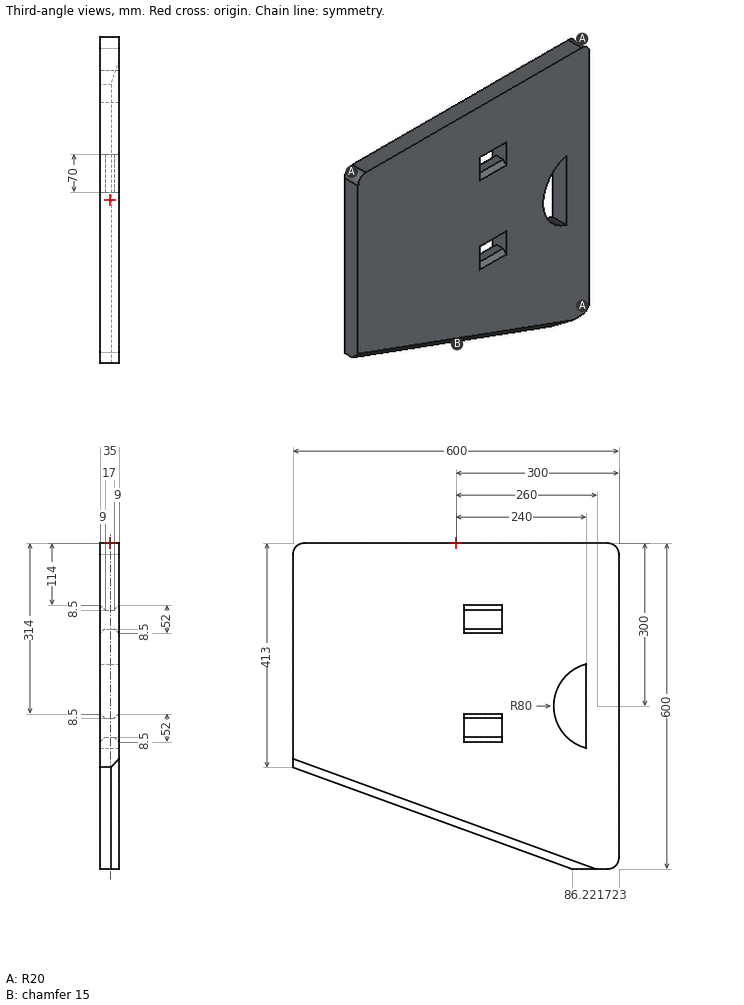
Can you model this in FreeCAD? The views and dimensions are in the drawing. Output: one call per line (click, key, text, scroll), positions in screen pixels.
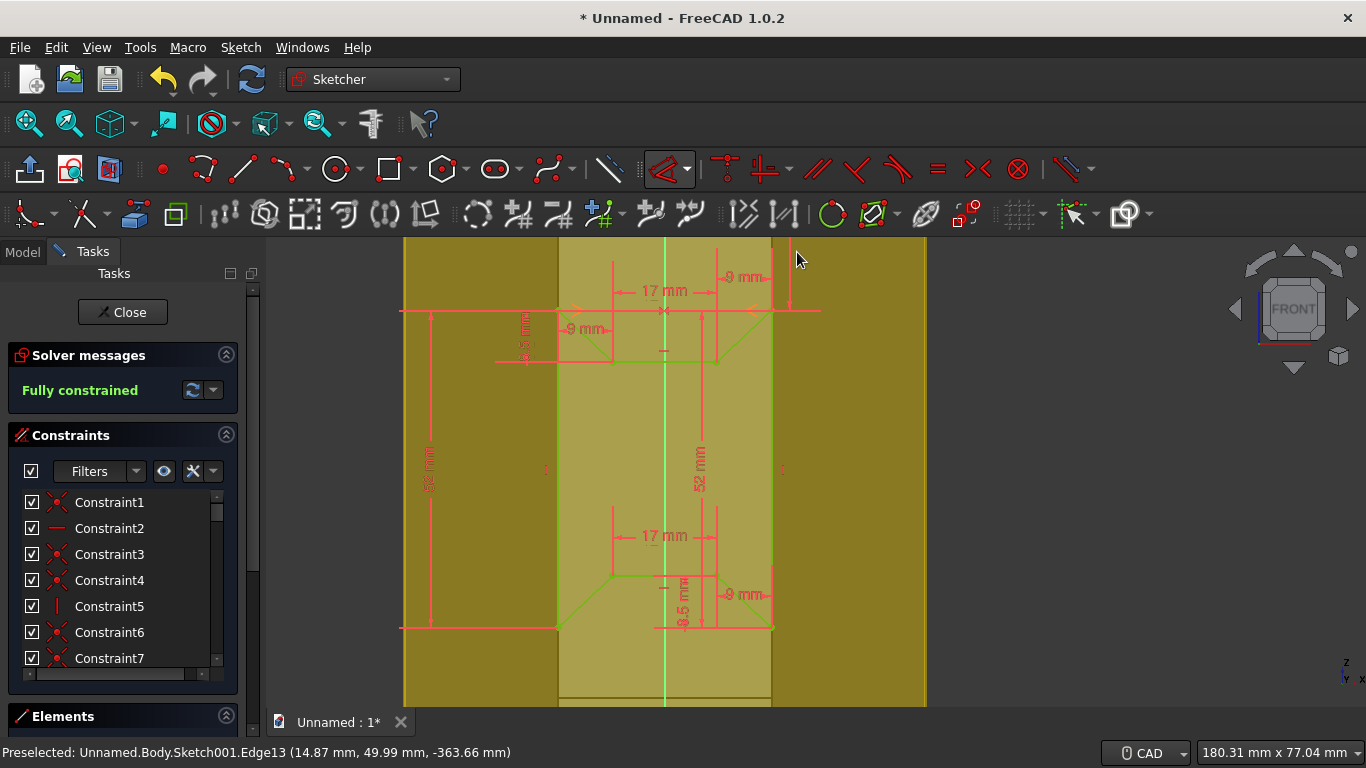
click(123, 312)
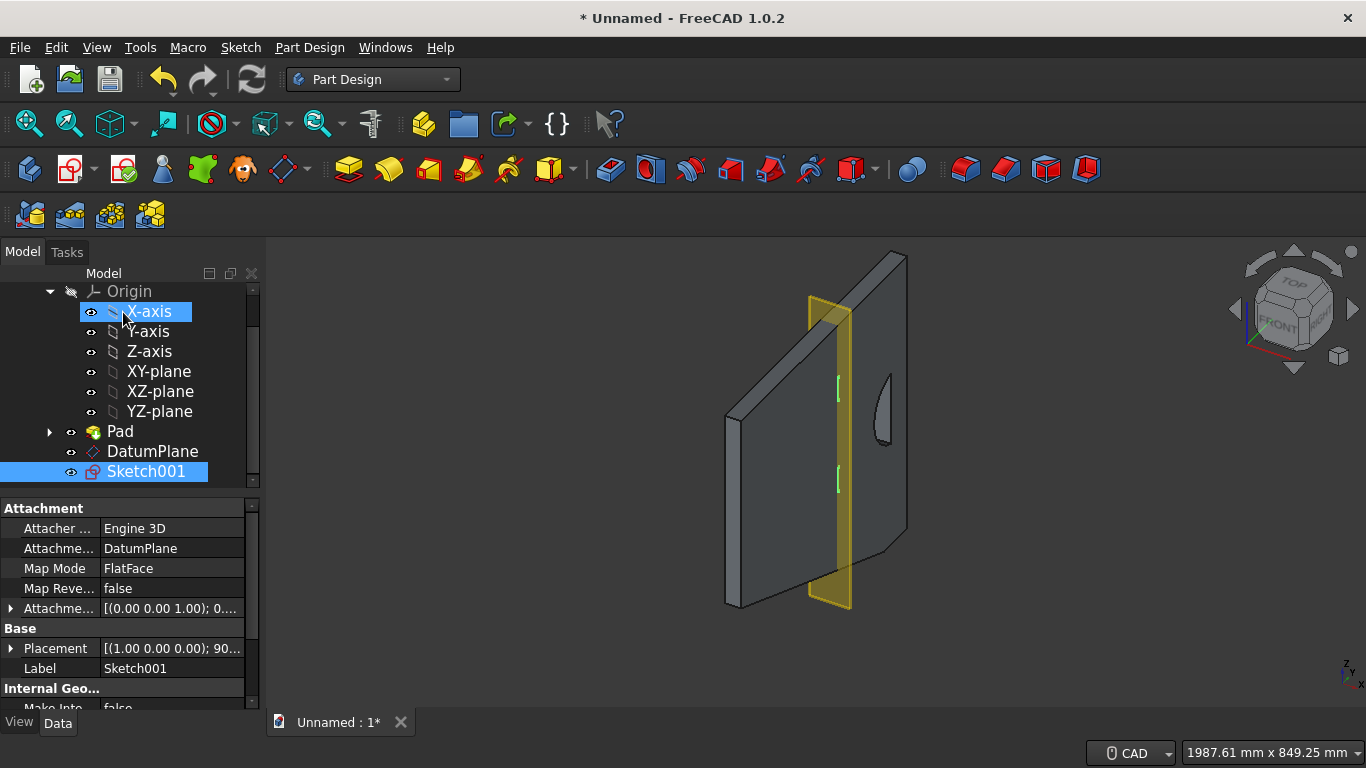
click(612, 170)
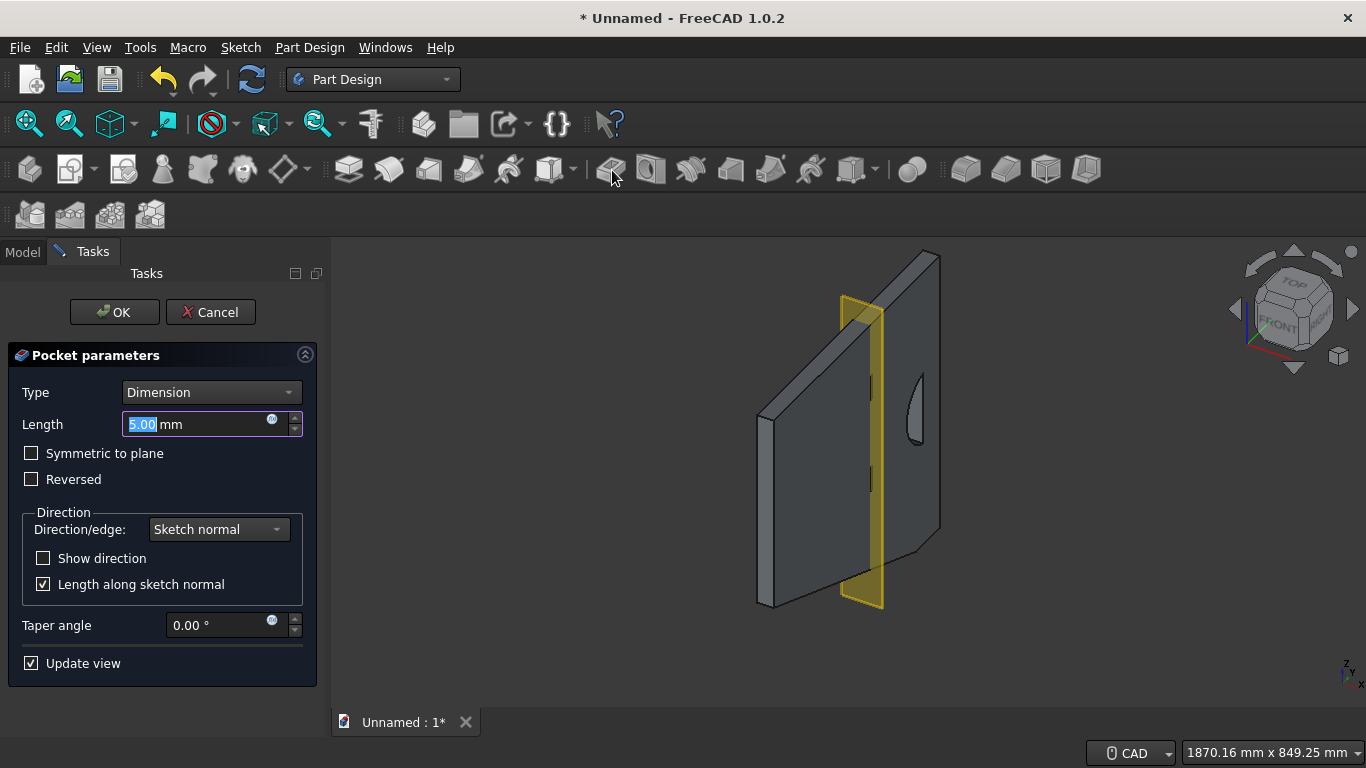
text(70)
key(Tab)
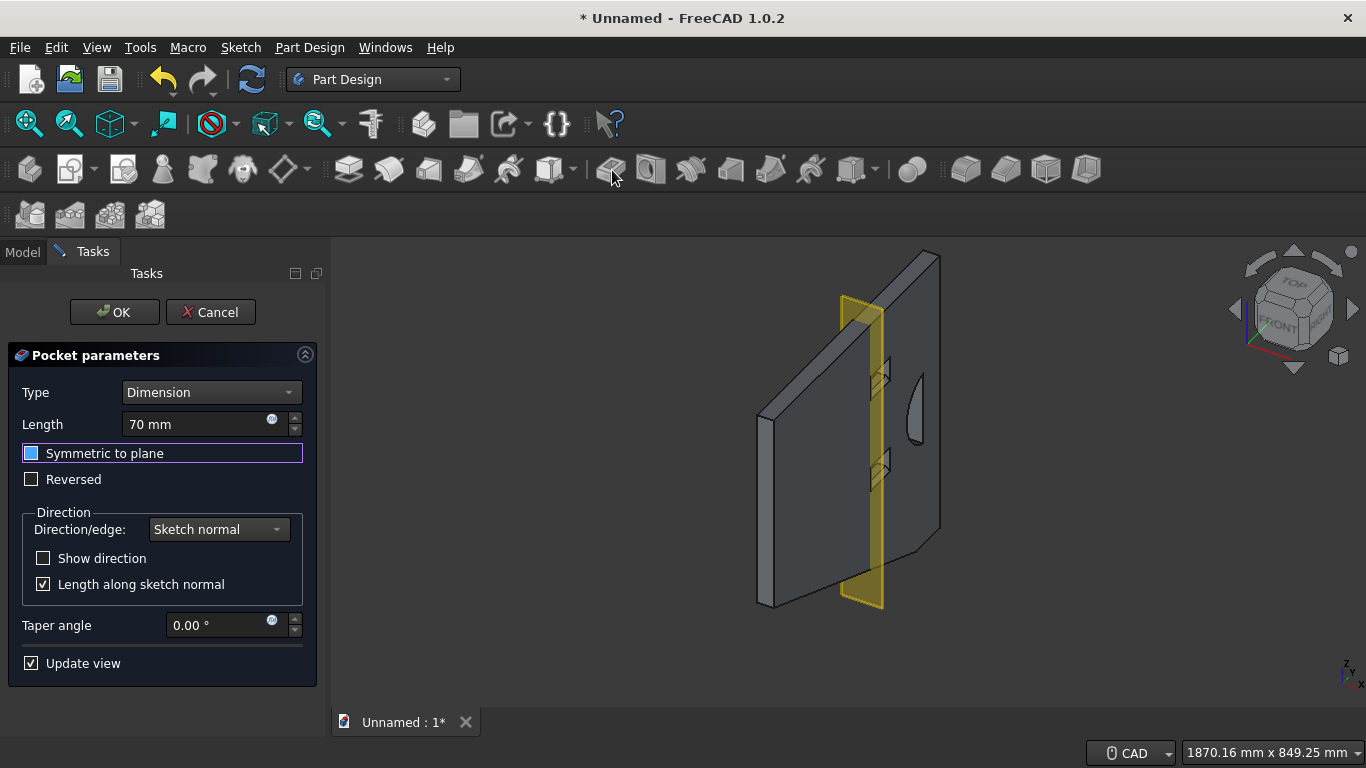
click(30, 453)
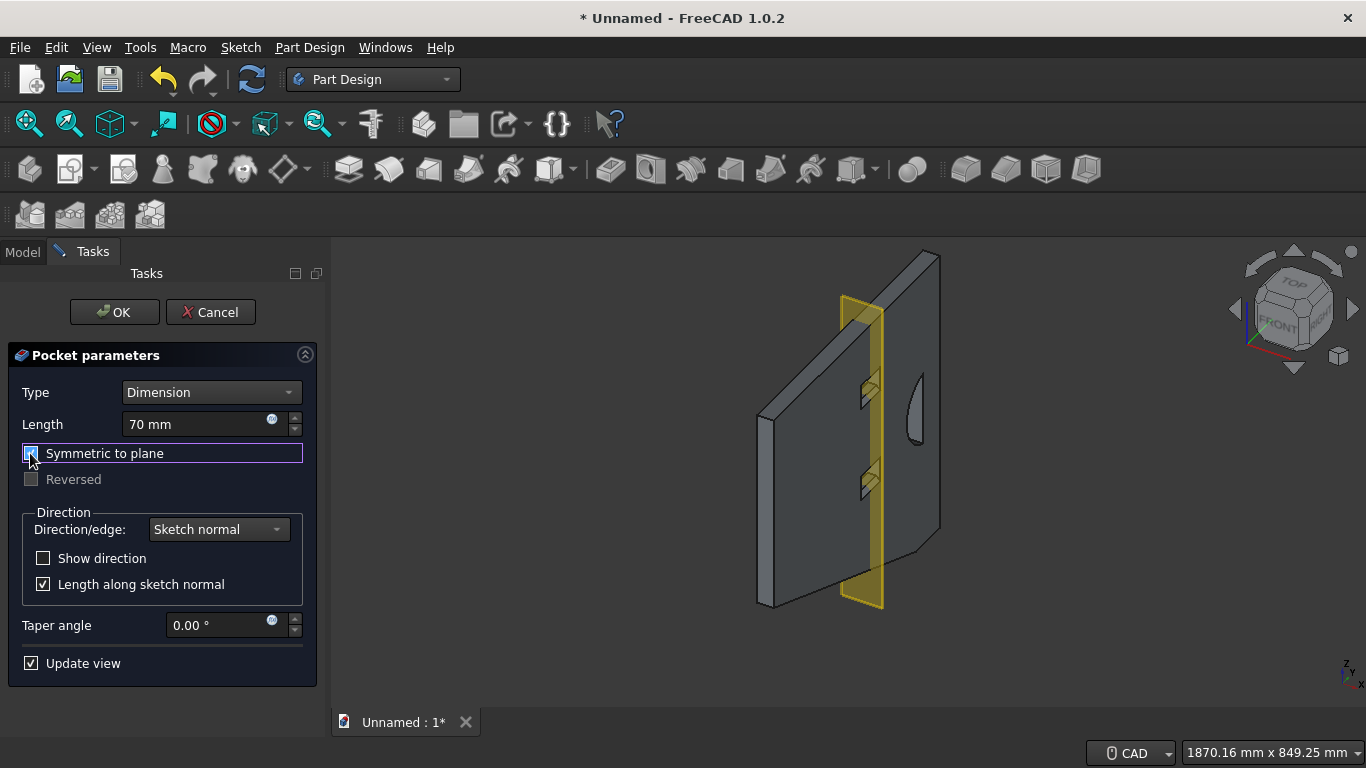
click(115, 312)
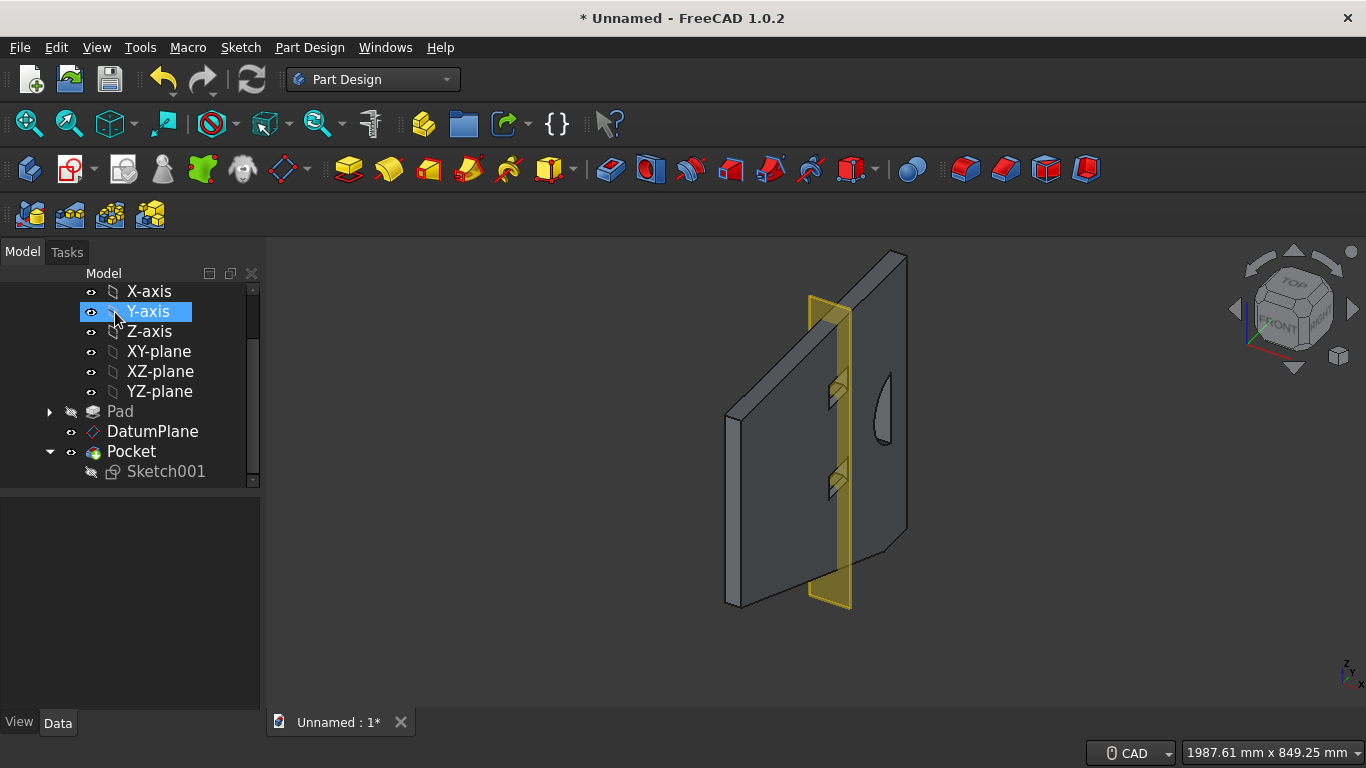
click(116, 432)
key(space)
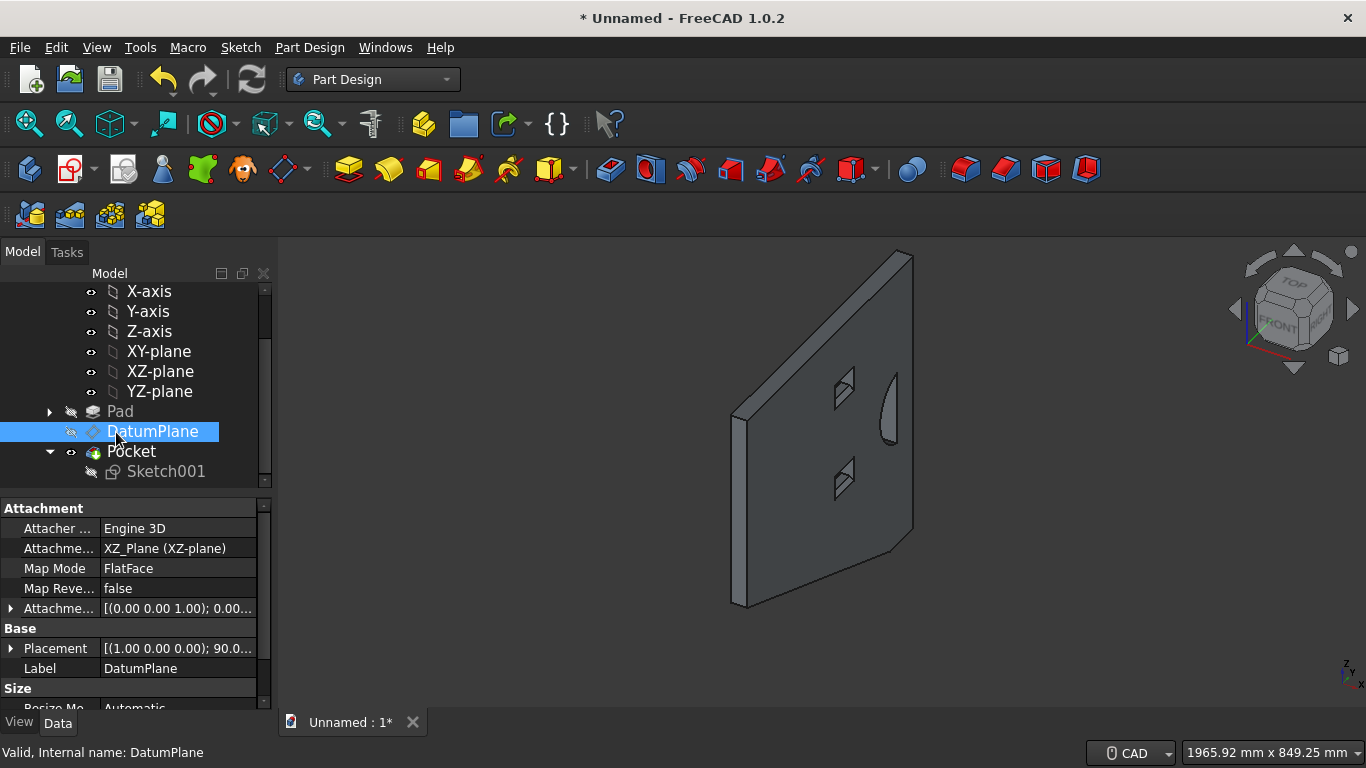
click(739, 417)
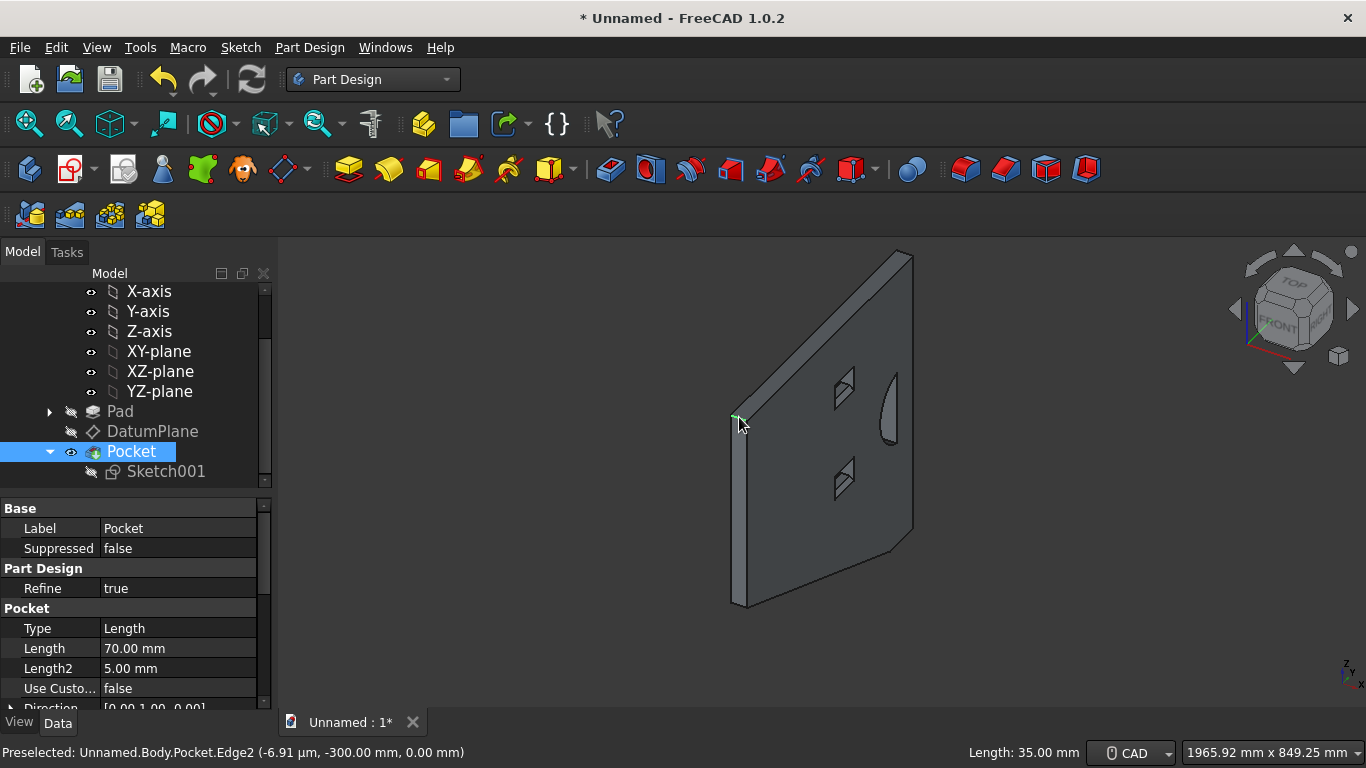
key(0)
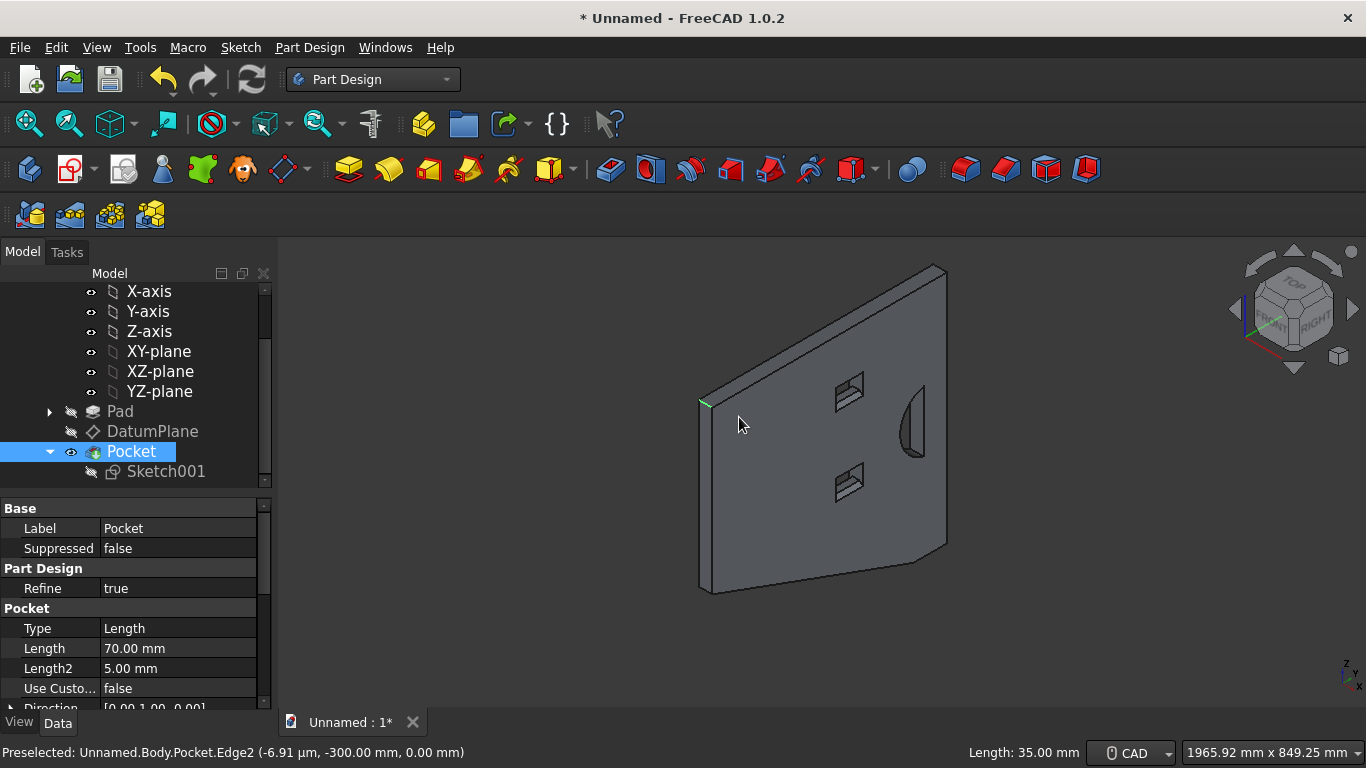
scroll(940, 267, up, 4)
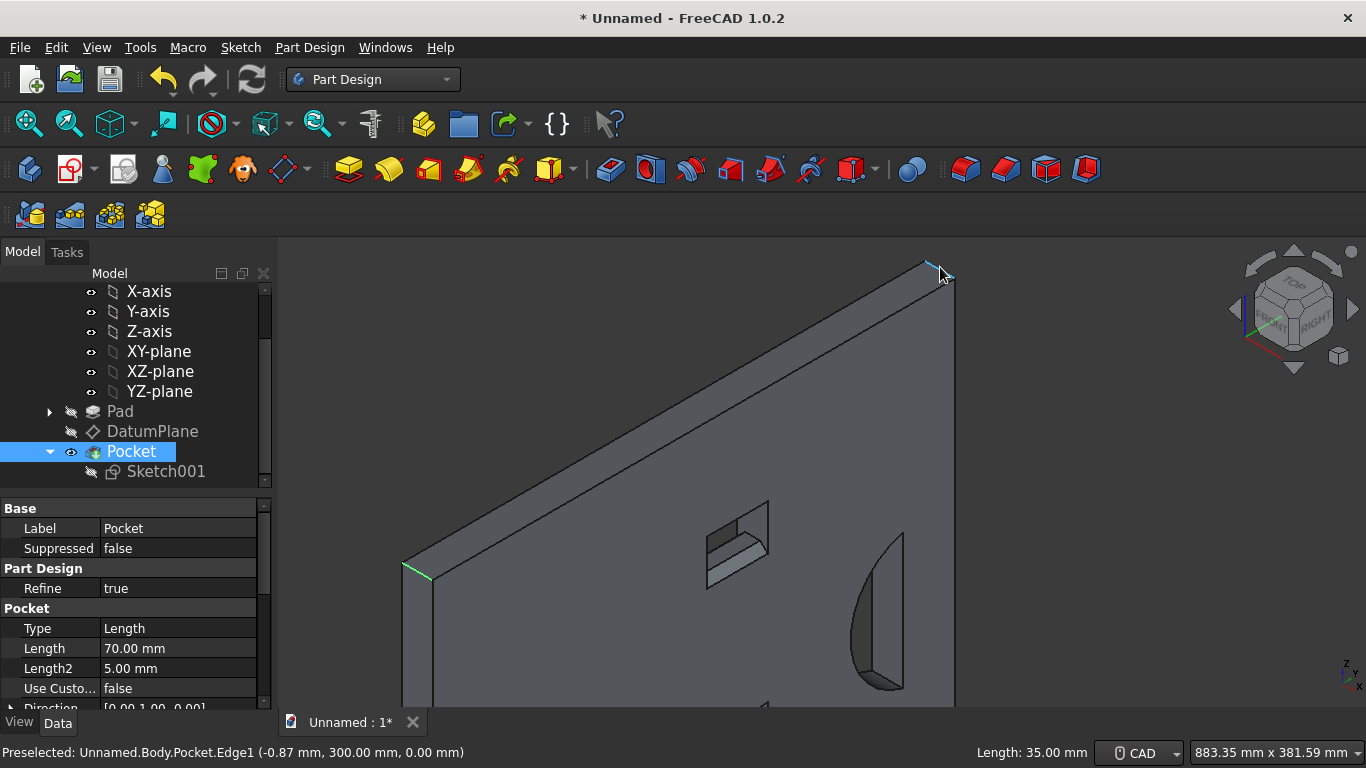
click(30, 124)